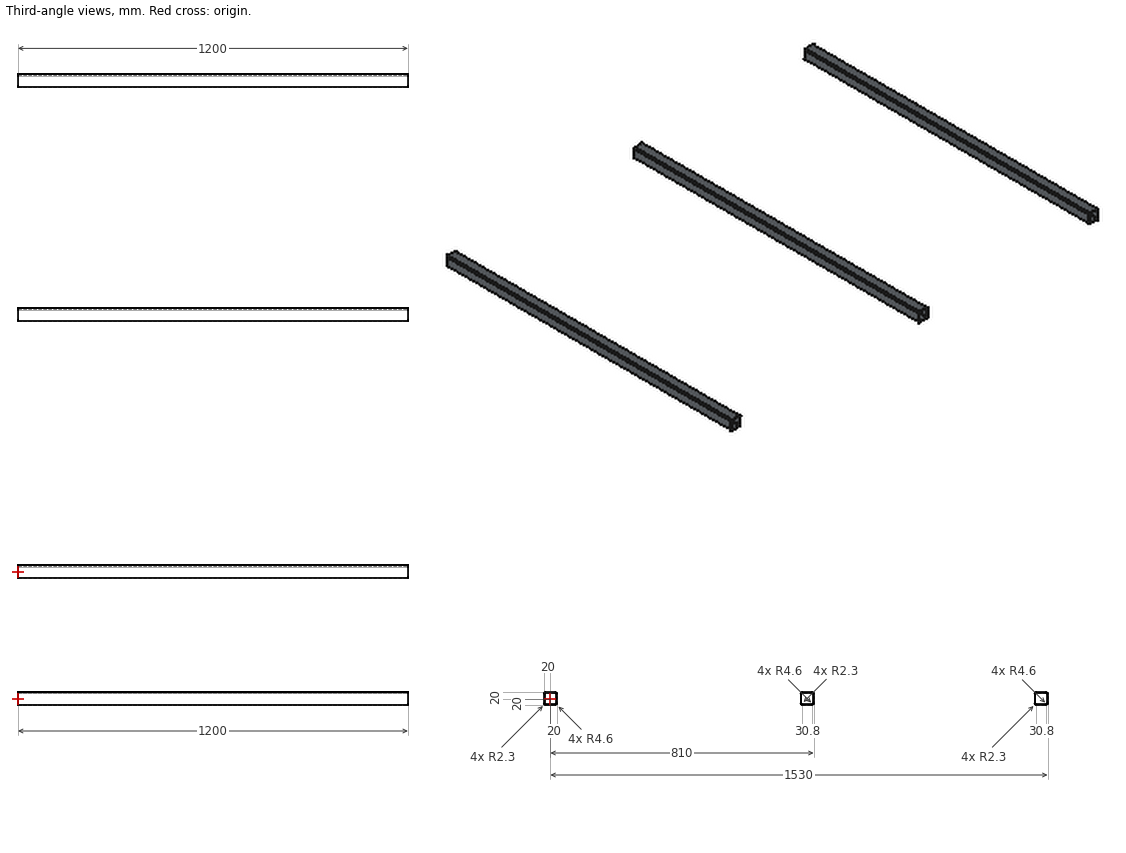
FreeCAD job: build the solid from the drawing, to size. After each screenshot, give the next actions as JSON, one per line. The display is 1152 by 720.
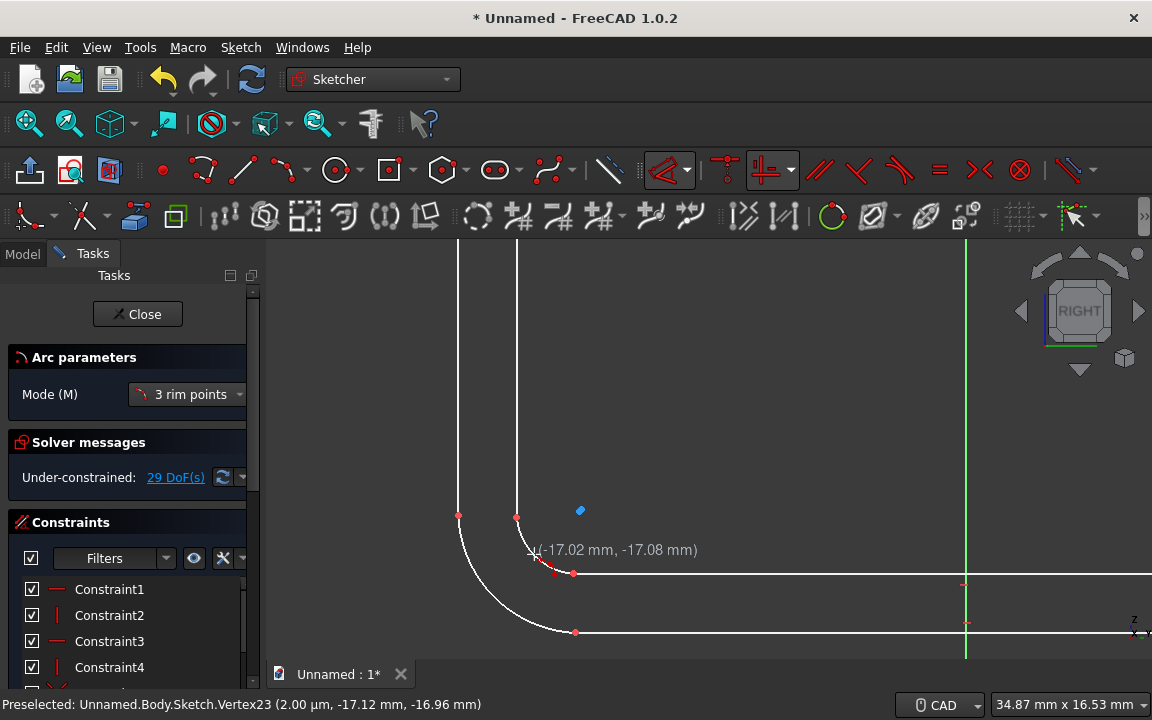
{"action": "scroll", "coordinate": [534, 556], "scroll_direction": "down", "scroll_amount": 7}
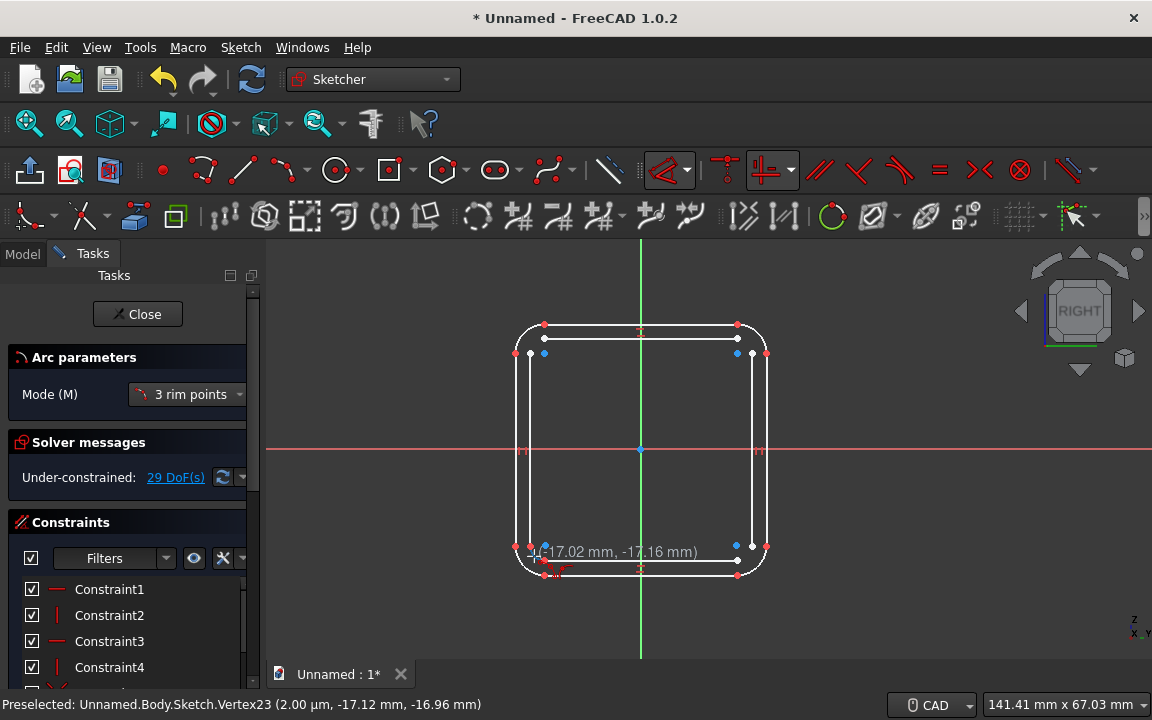
{"action": "left_click", "coordinate": [530, 354]}
{"action": "left_click", "coordinate": [544, 339]}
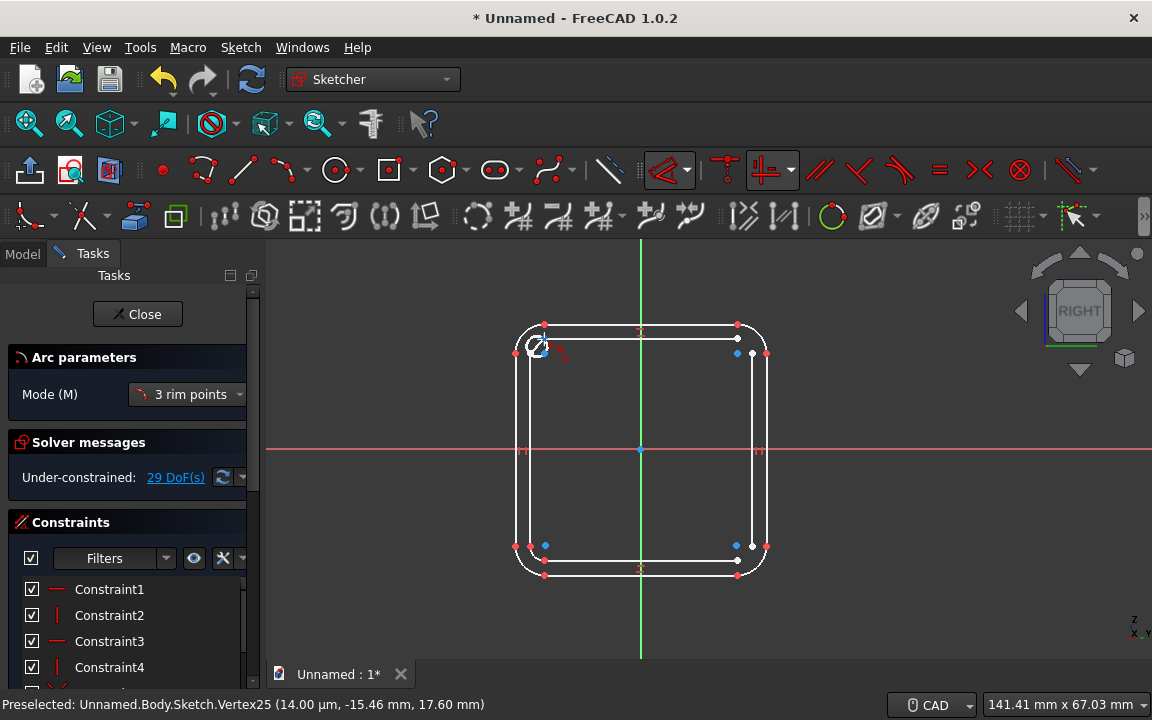
{"action": "scroll", "coordinate": [534, 343], "scroll_direction": "up", "scroll_amount": 7}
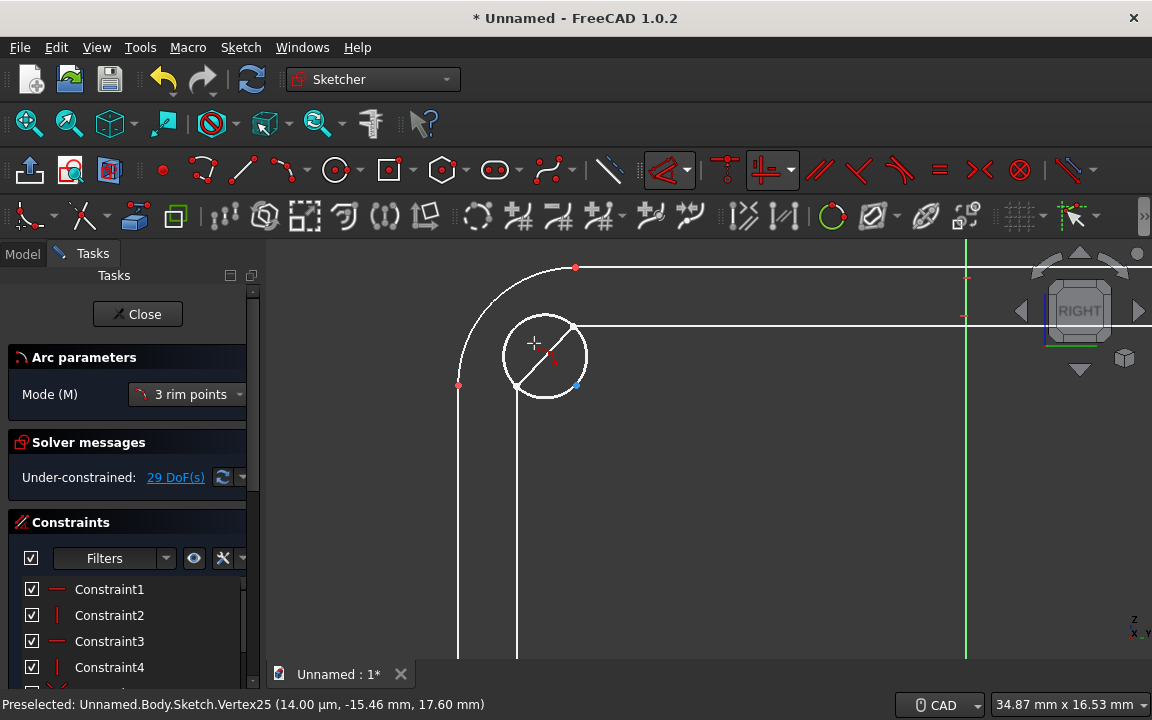
{"action": "left_click", "coordinate": [534, 341]}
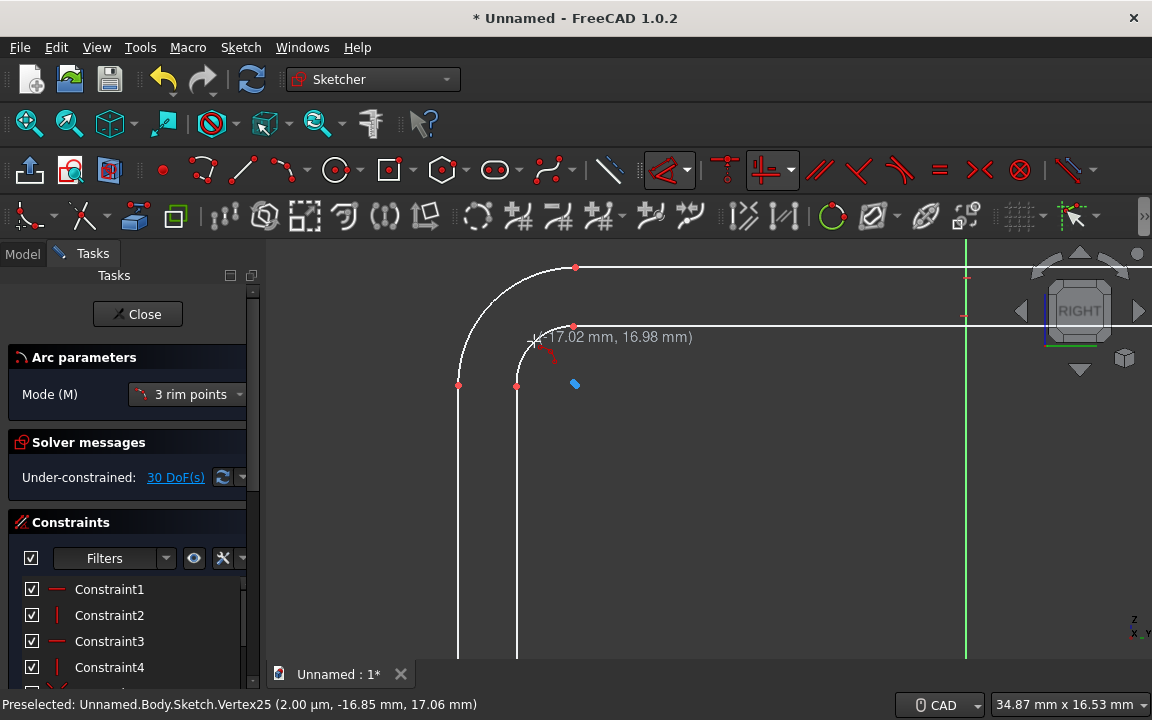
{"action": "scroll", "coordinate": [534, 343], "scroll_direction": "down", "scroll_amount": 7}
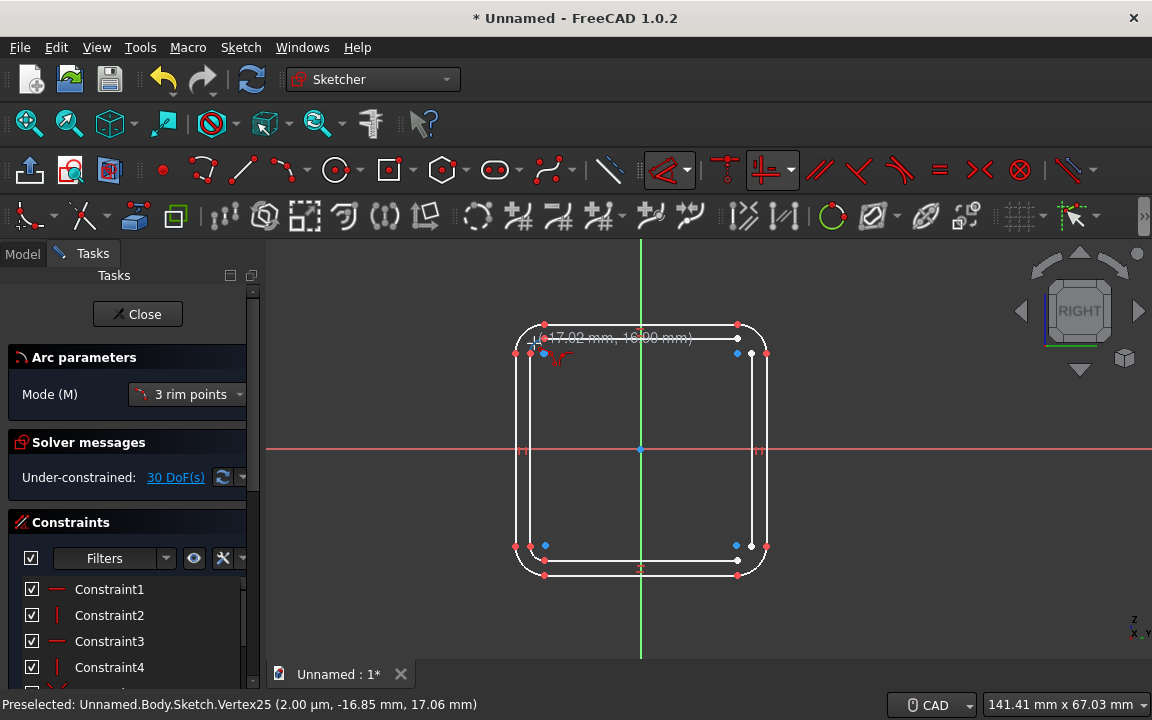
{"action": "left_click", "coordinate": [737, 339]}
{"action": "left_click", "coordinate": [752, 354]}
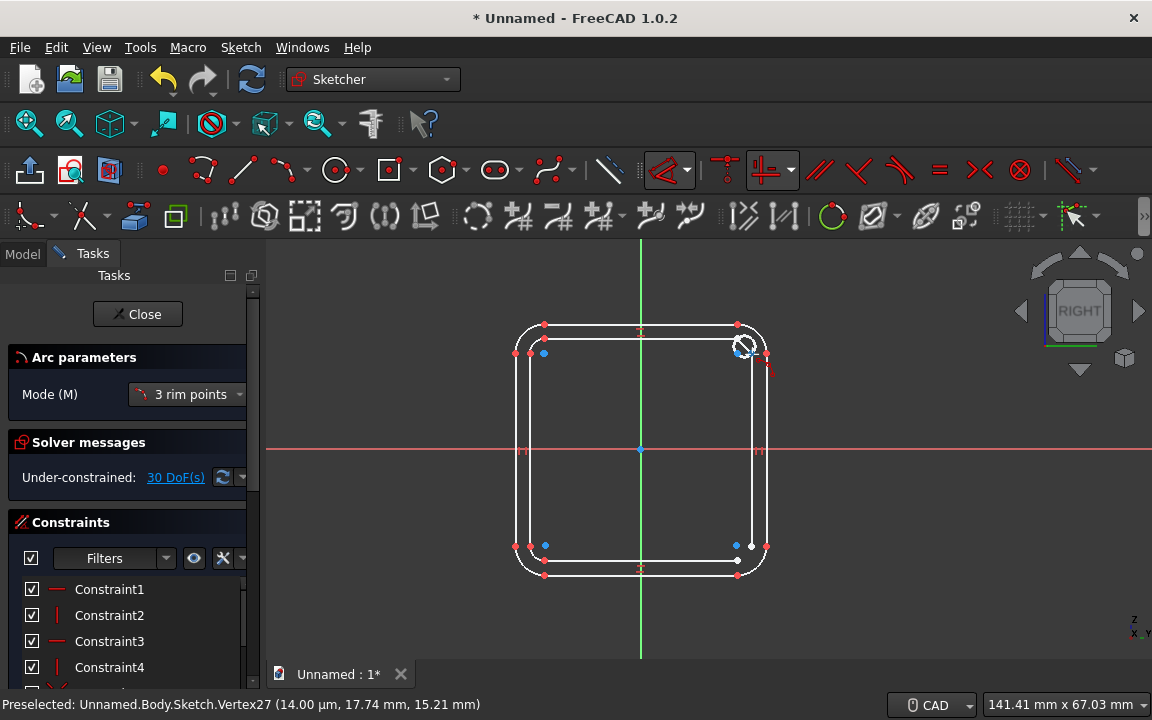
{"action": "scroll", "coordinate": [748, 343], "scroll_direction": "up", "scroll_amount": 7}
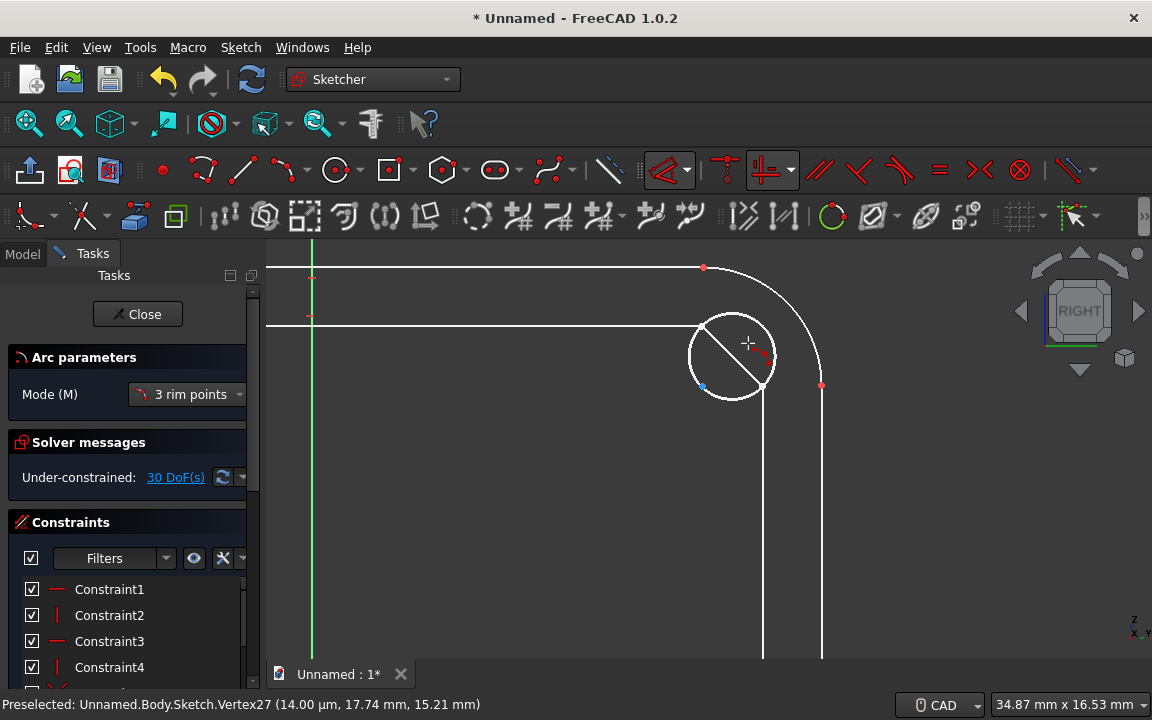
{"action": "left_click", "coordinate": [744, 341]}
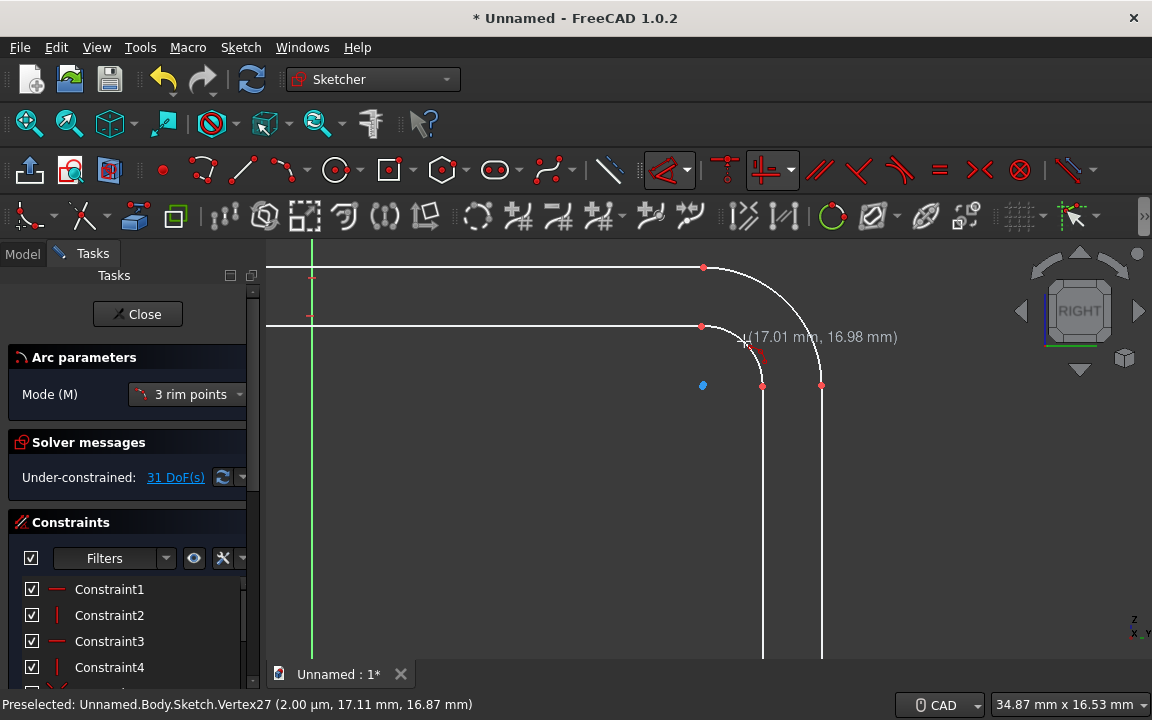
{"action": "scroll", "coordinate": [748, 343], "scroll_direction": "down", "scroll_amount": 7}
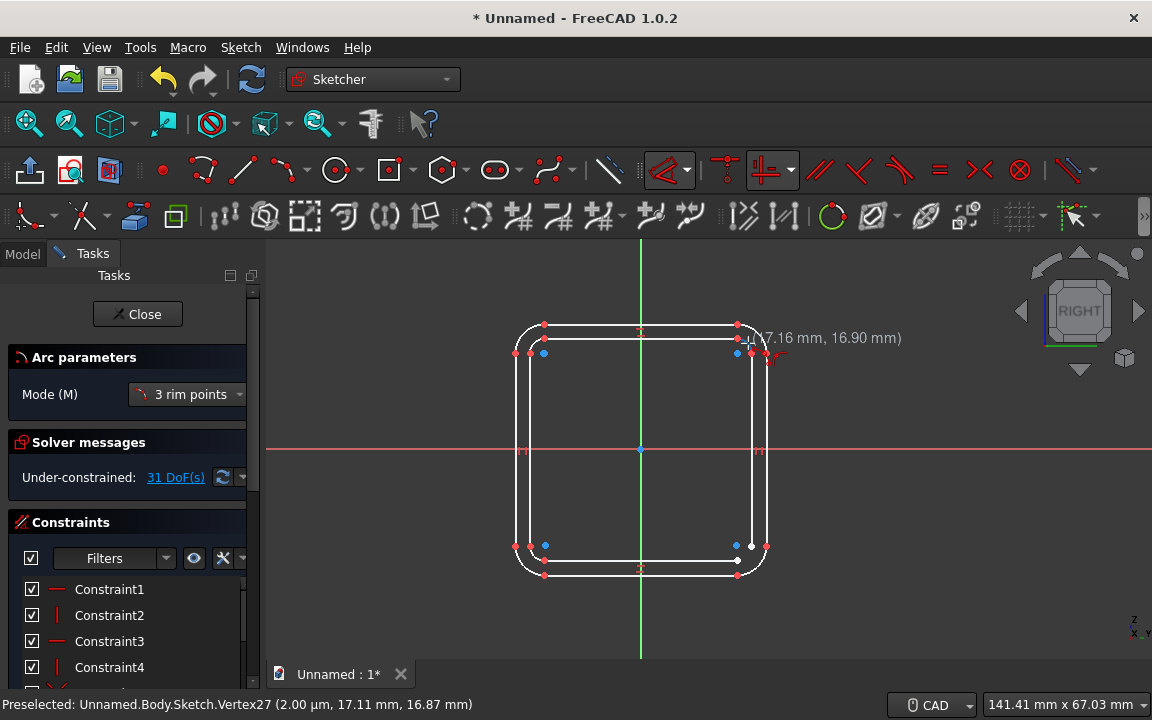
{"action": "left_click", "coordinate": [752, 547]}
{"action": "left_click", "coordinate": [737, 561]}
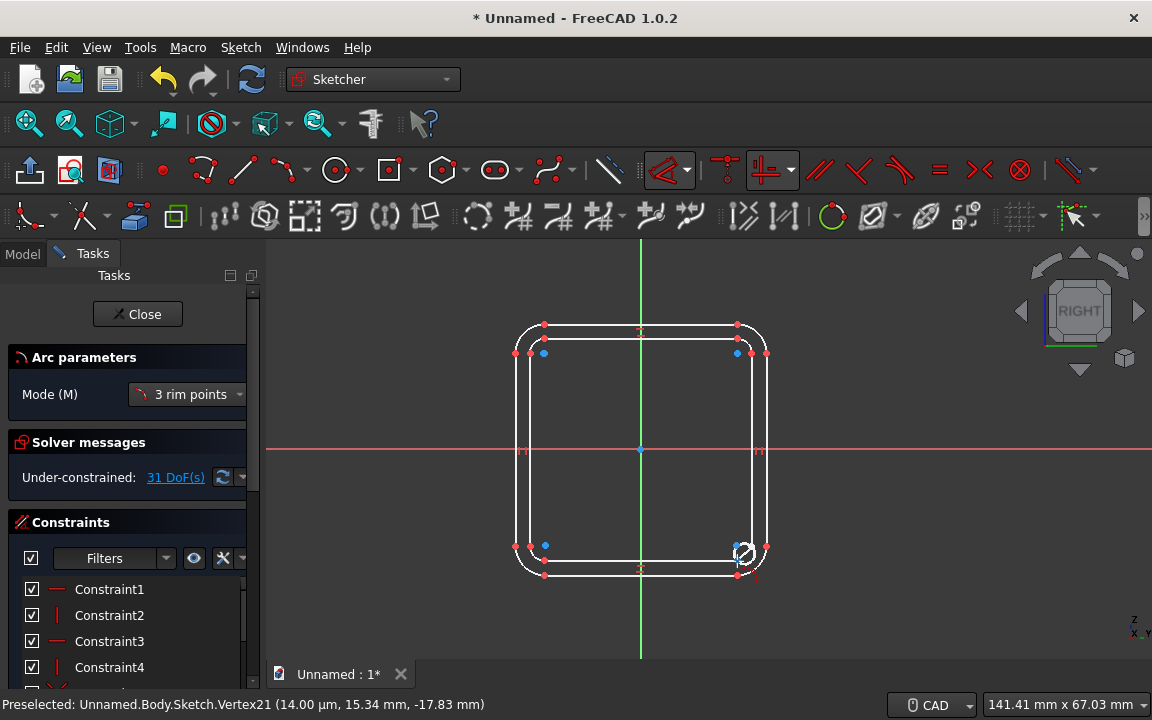
{"action": "scroll", "coordinate": [748, 556], "scroll_direction": "up", "scroll_amount": 7}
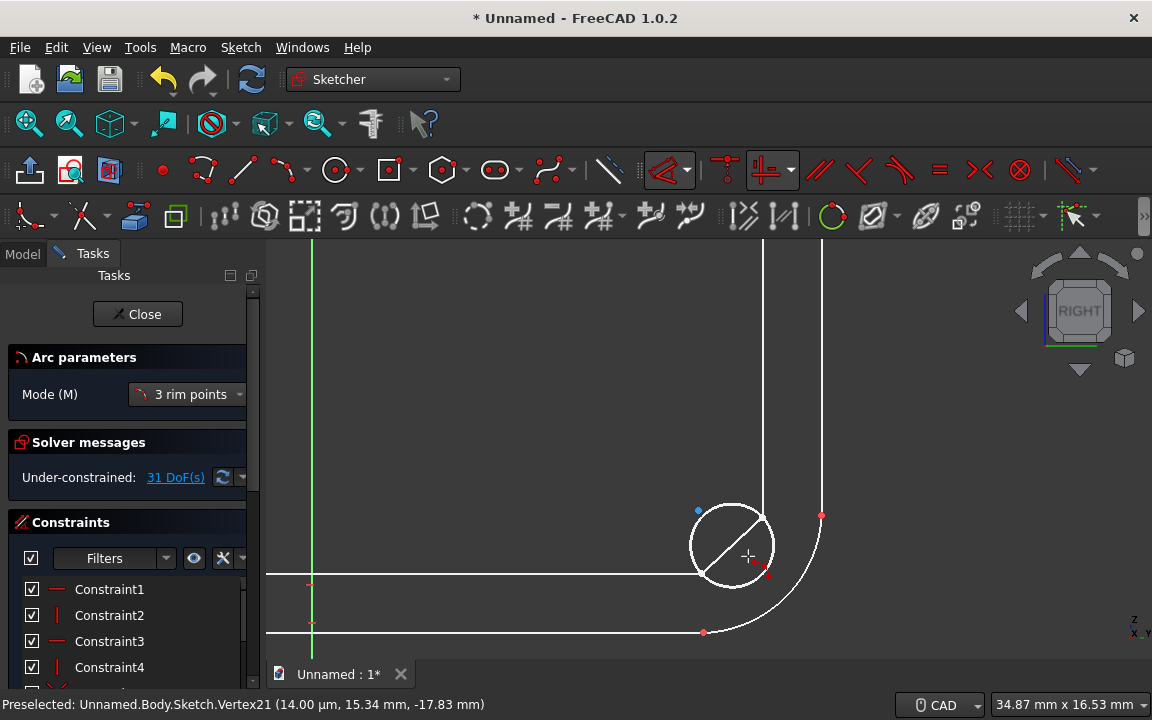
{"action": "left_click", "coordinate": [744, 554]}
{"action": "key", "text": "Escape"}